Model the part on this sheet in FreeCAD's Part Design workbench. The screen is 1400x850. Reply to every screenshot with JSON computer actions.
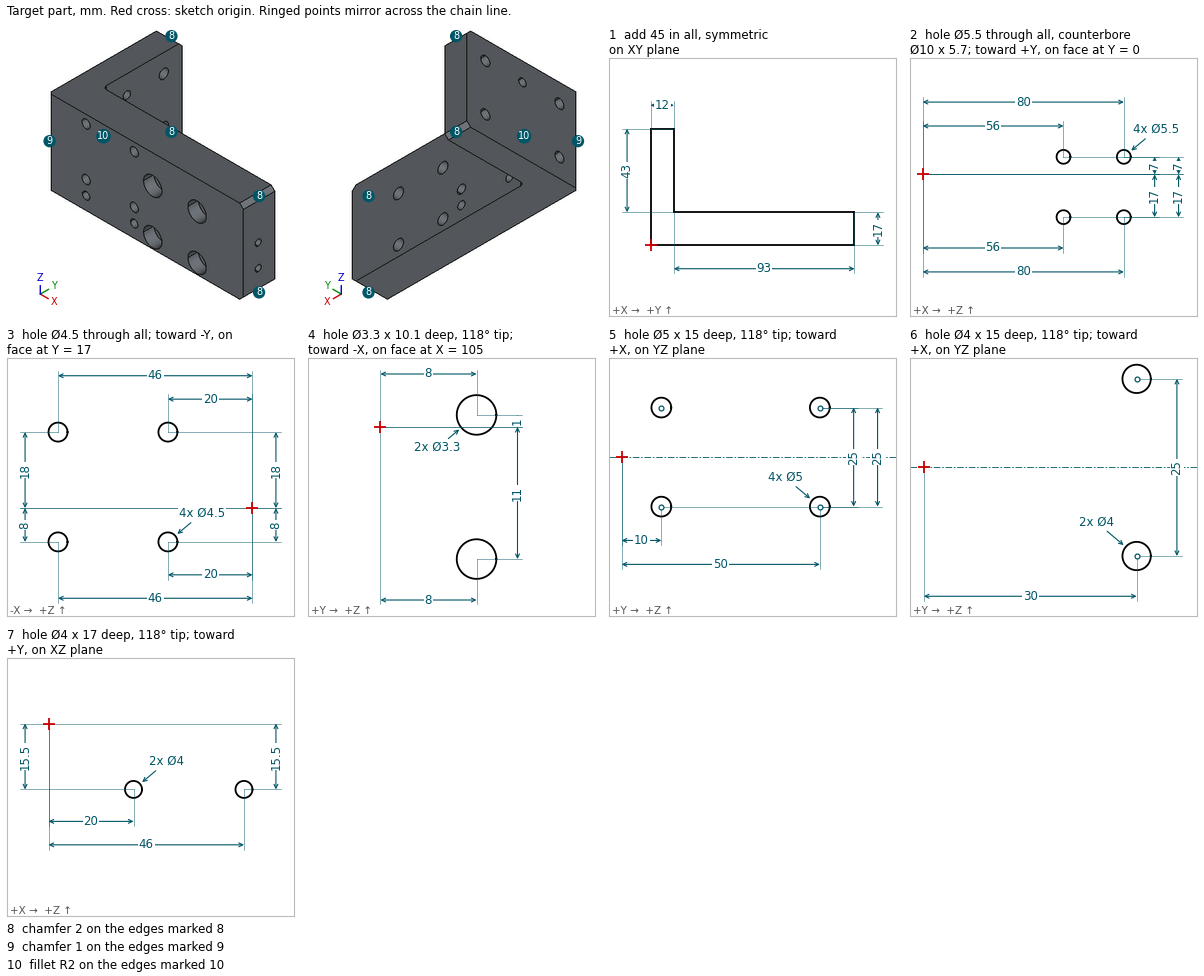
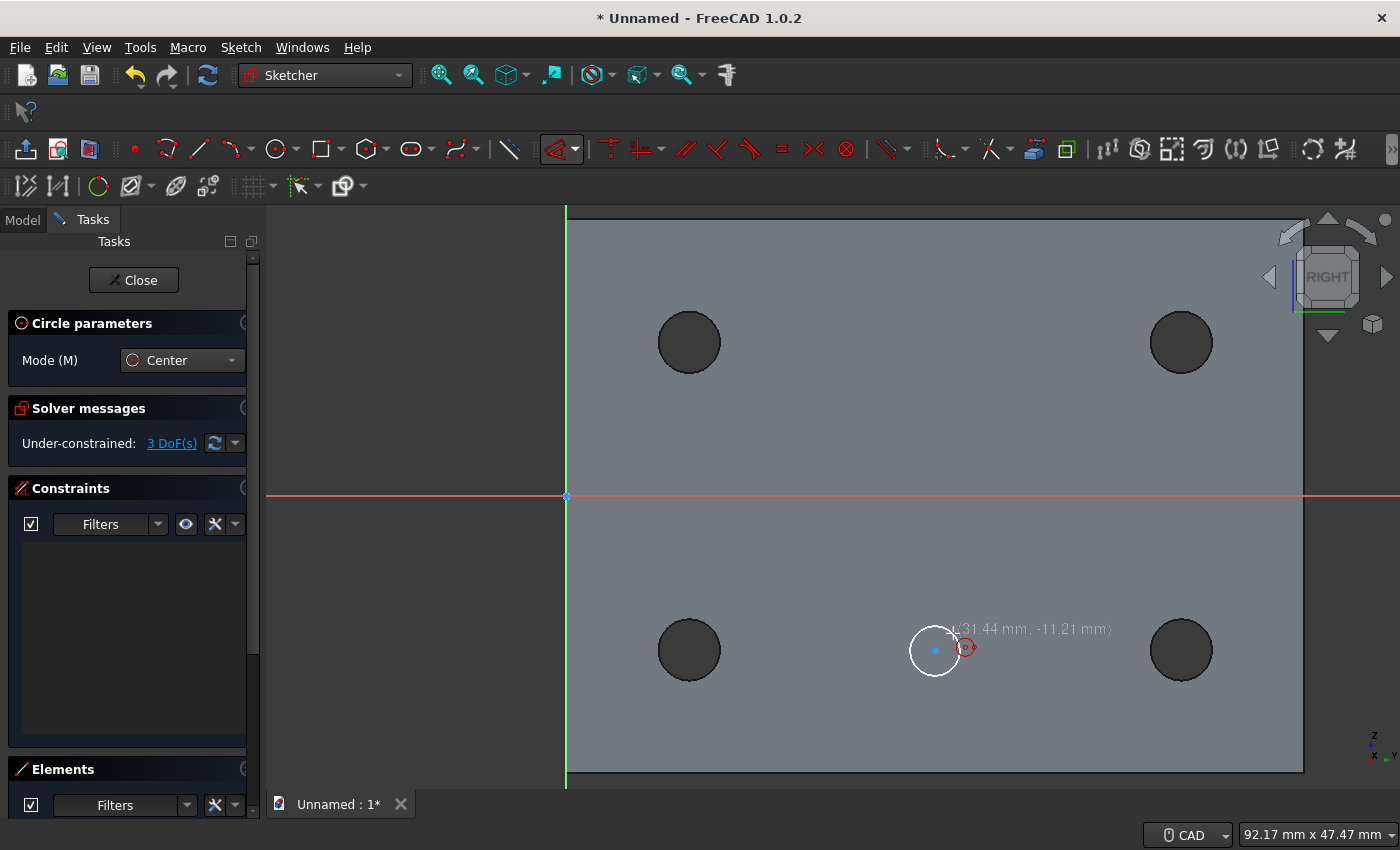
{"action": "left_click", "coordinate": [935, 342]}
{"action": "left_click", "coordinate": [953, 325]}
{"action": "key", "text": "Escape"}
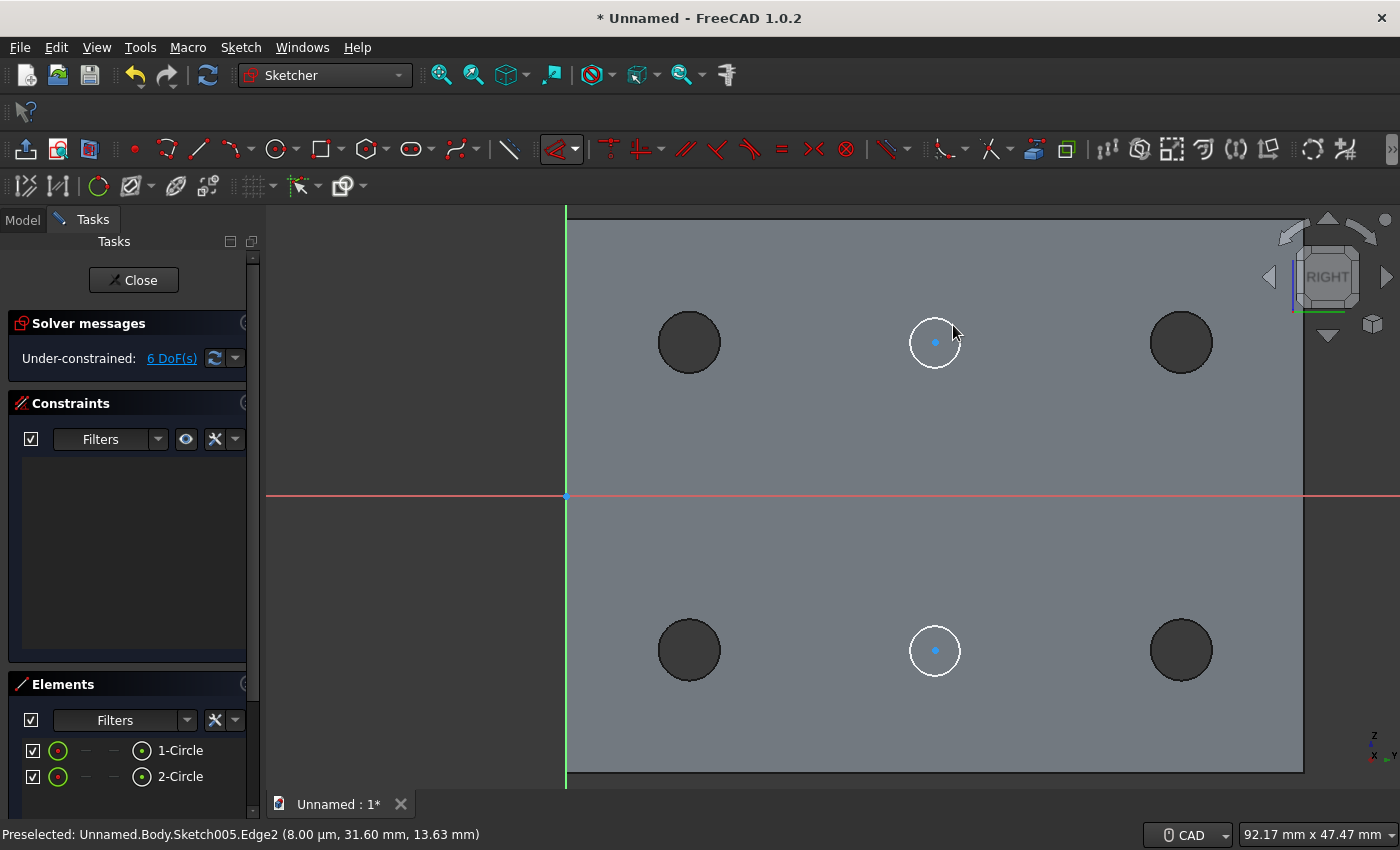
{"action": "left_click", "coordinate": [952, 633]}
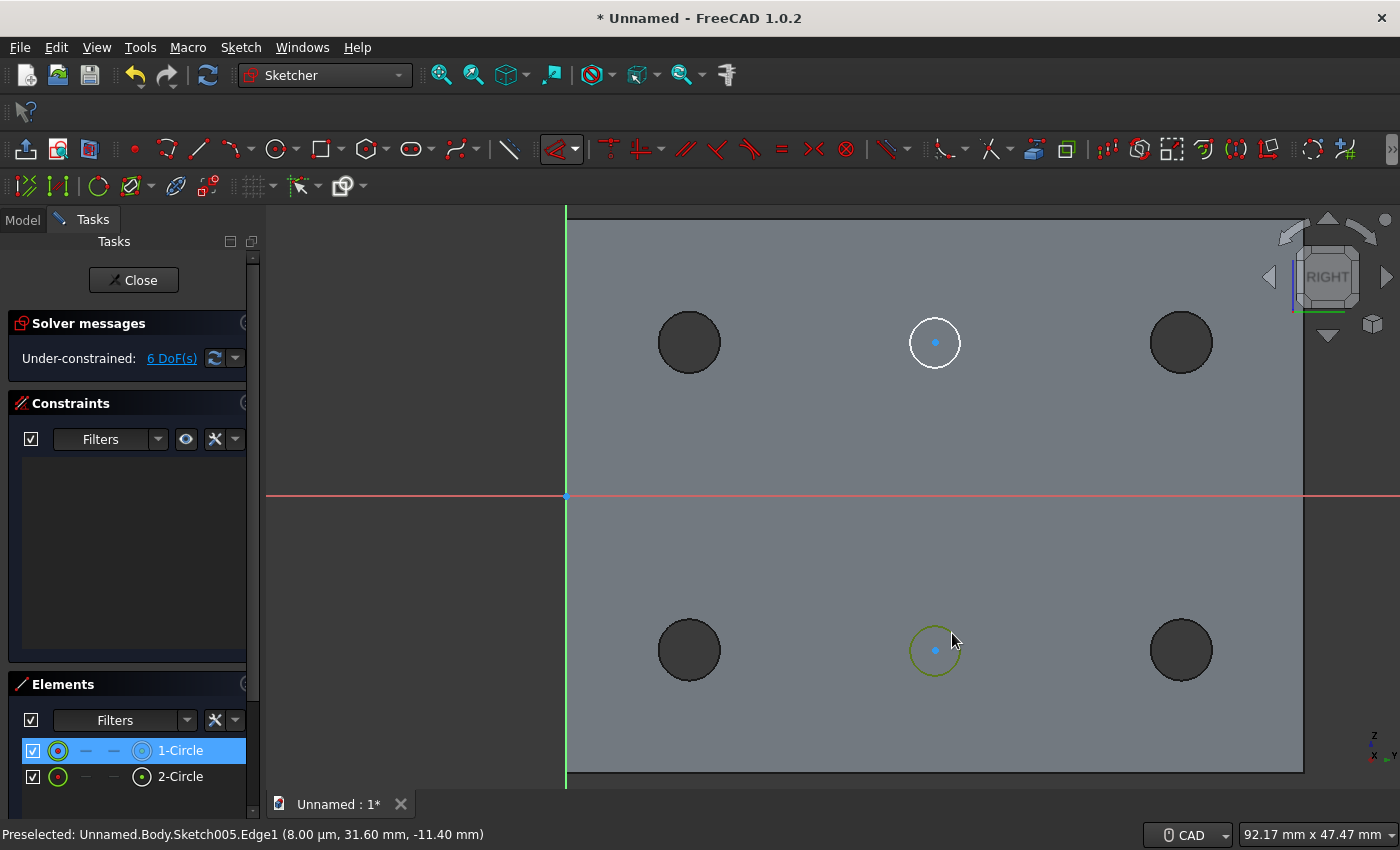
{"action": "left_click", "coordinate": [952, 325]}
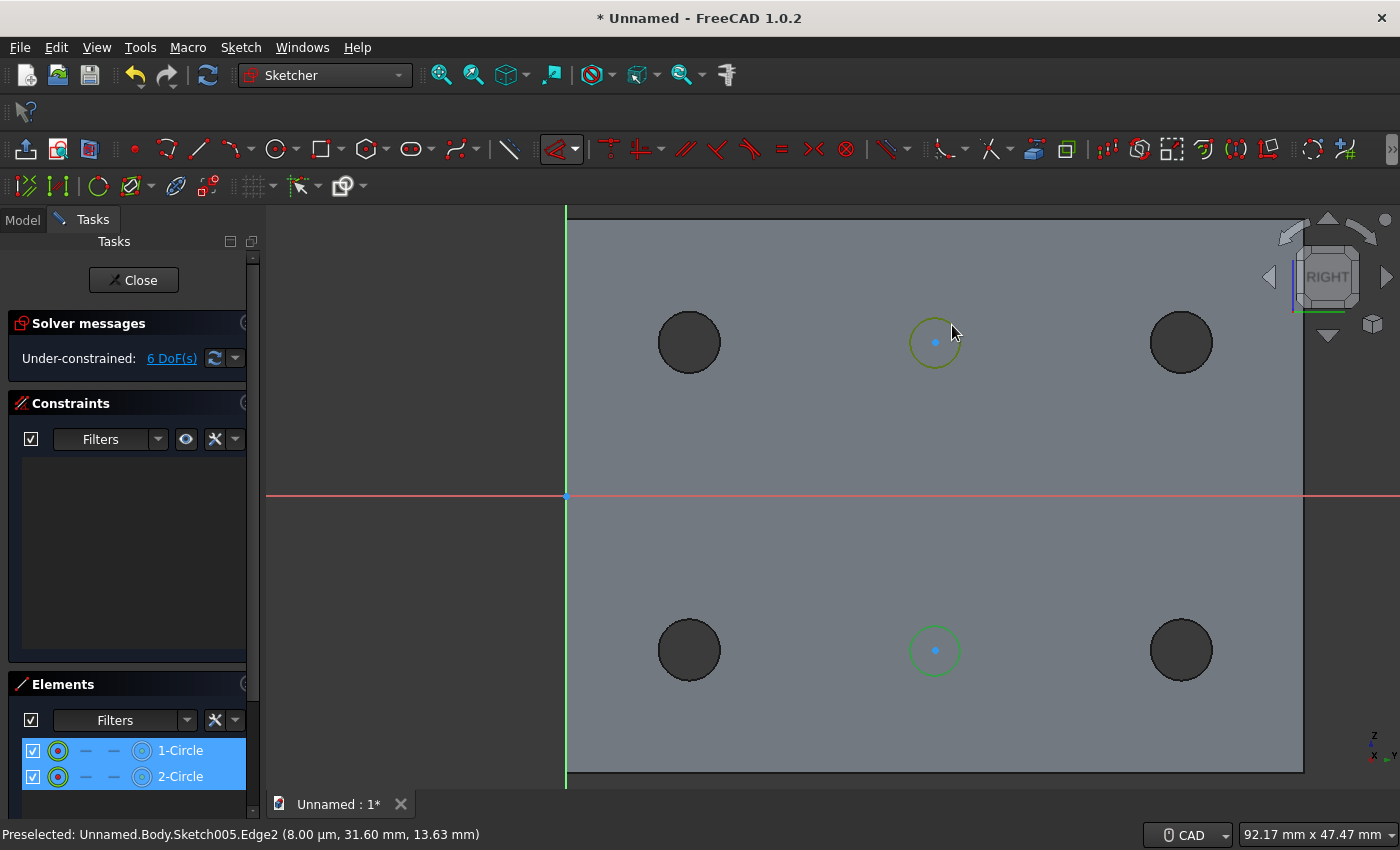
{"action": "key", "text": "e"}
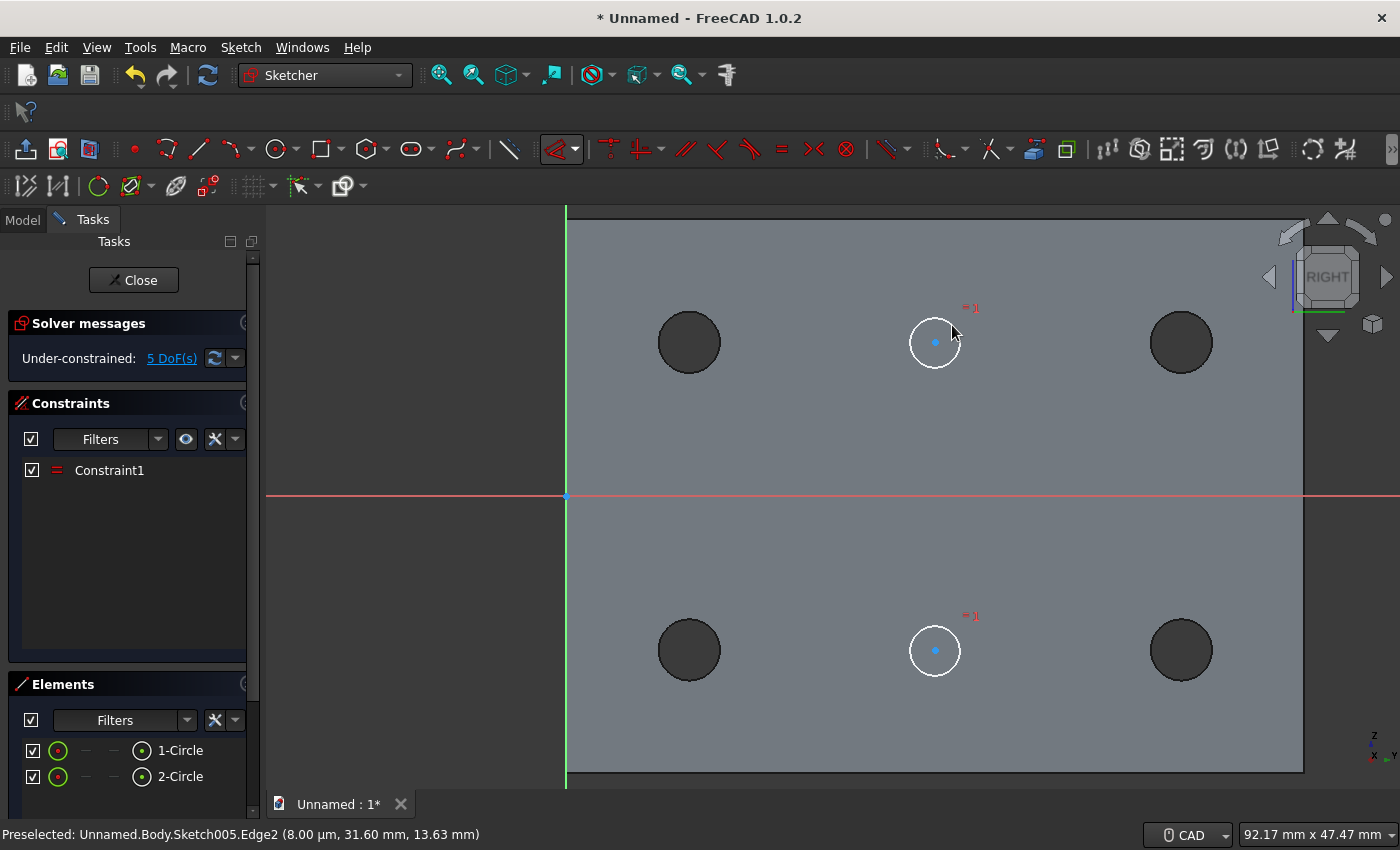
{"action": "left_click", "coordinate": [935, 651]}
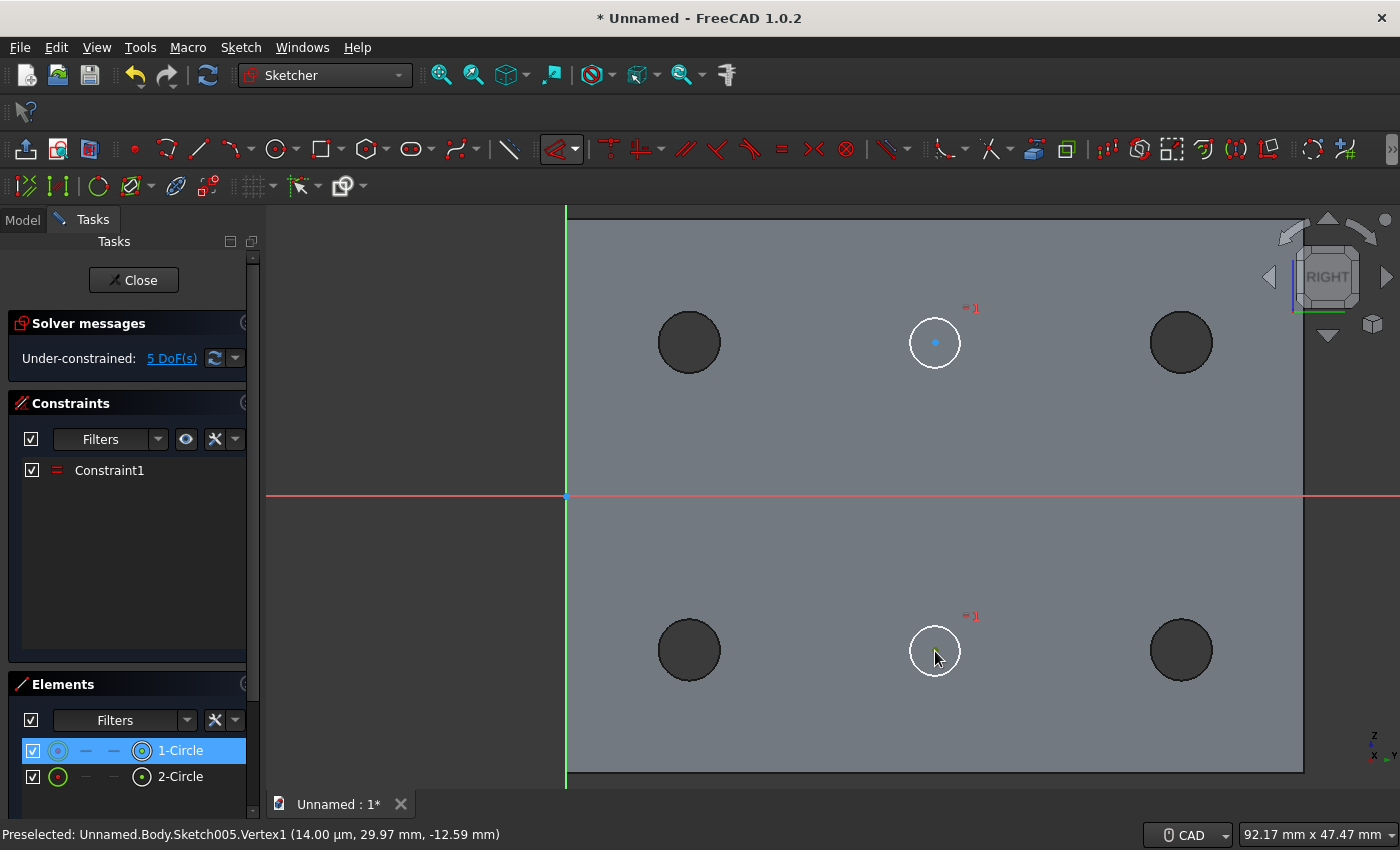
{"action": "left_click", "coordinate": [935, 343]}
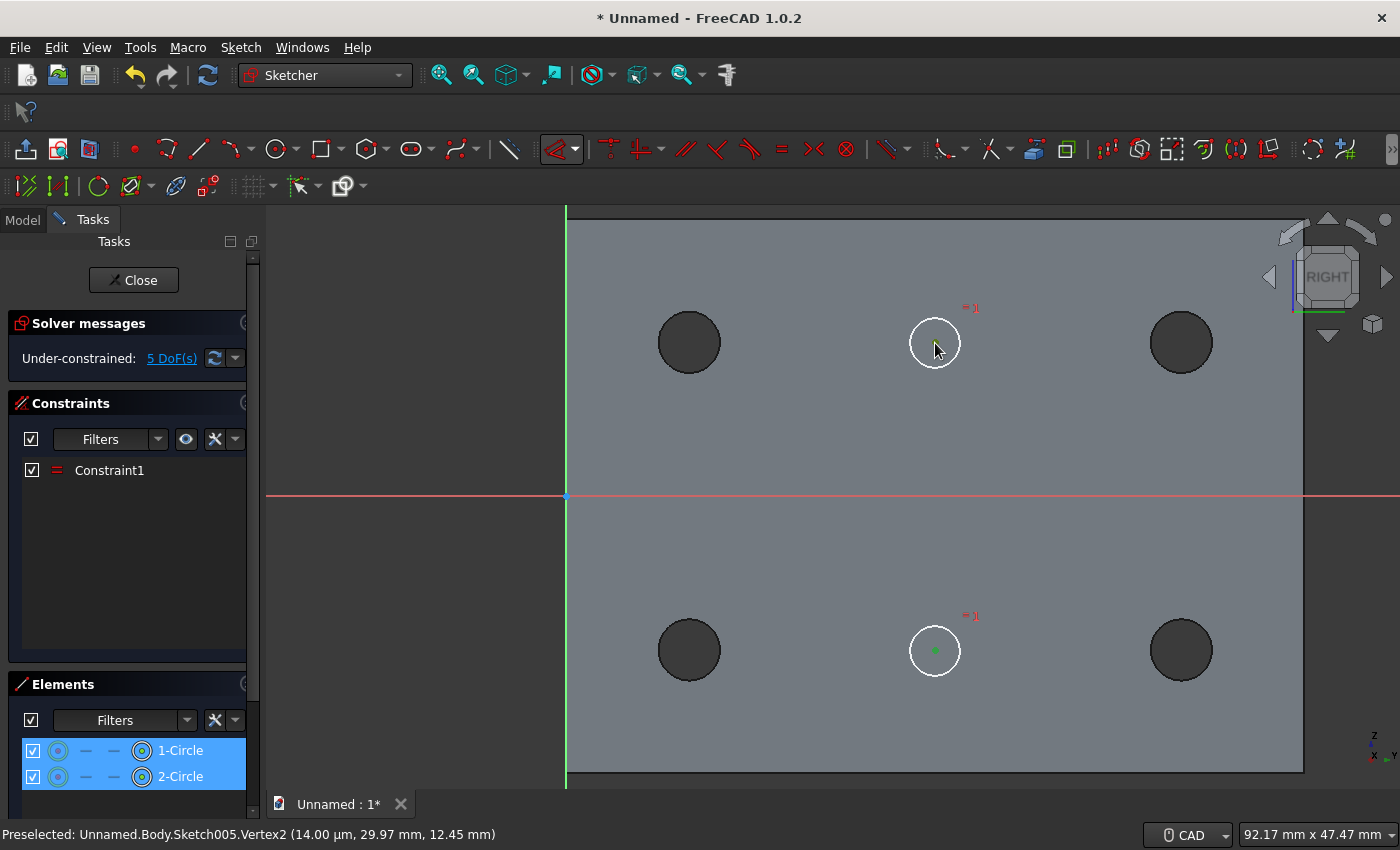
{"action": "left_click", "coordinate": [361, 496]}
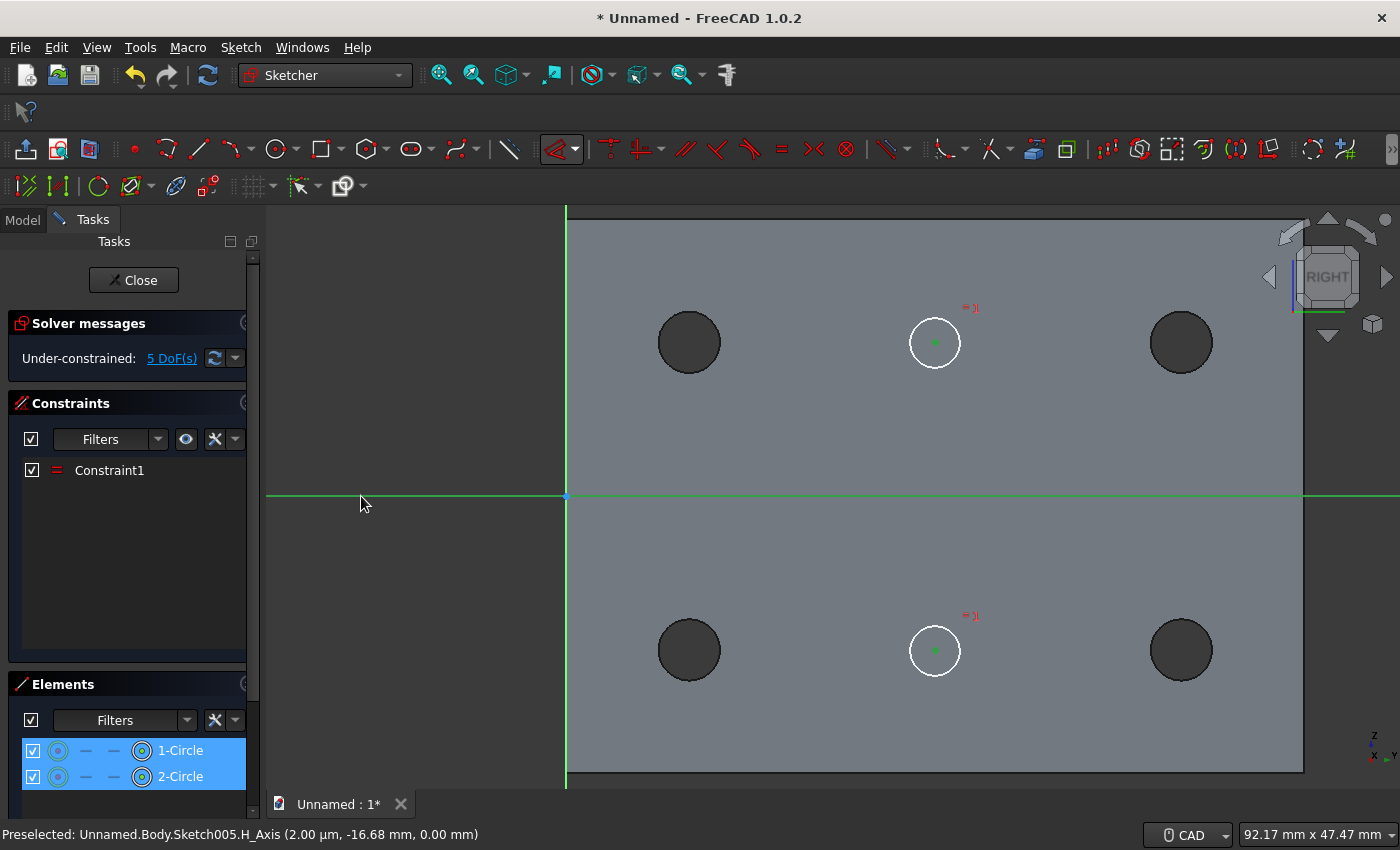
{"action": "left_click", "coordinate": [814, 150]}